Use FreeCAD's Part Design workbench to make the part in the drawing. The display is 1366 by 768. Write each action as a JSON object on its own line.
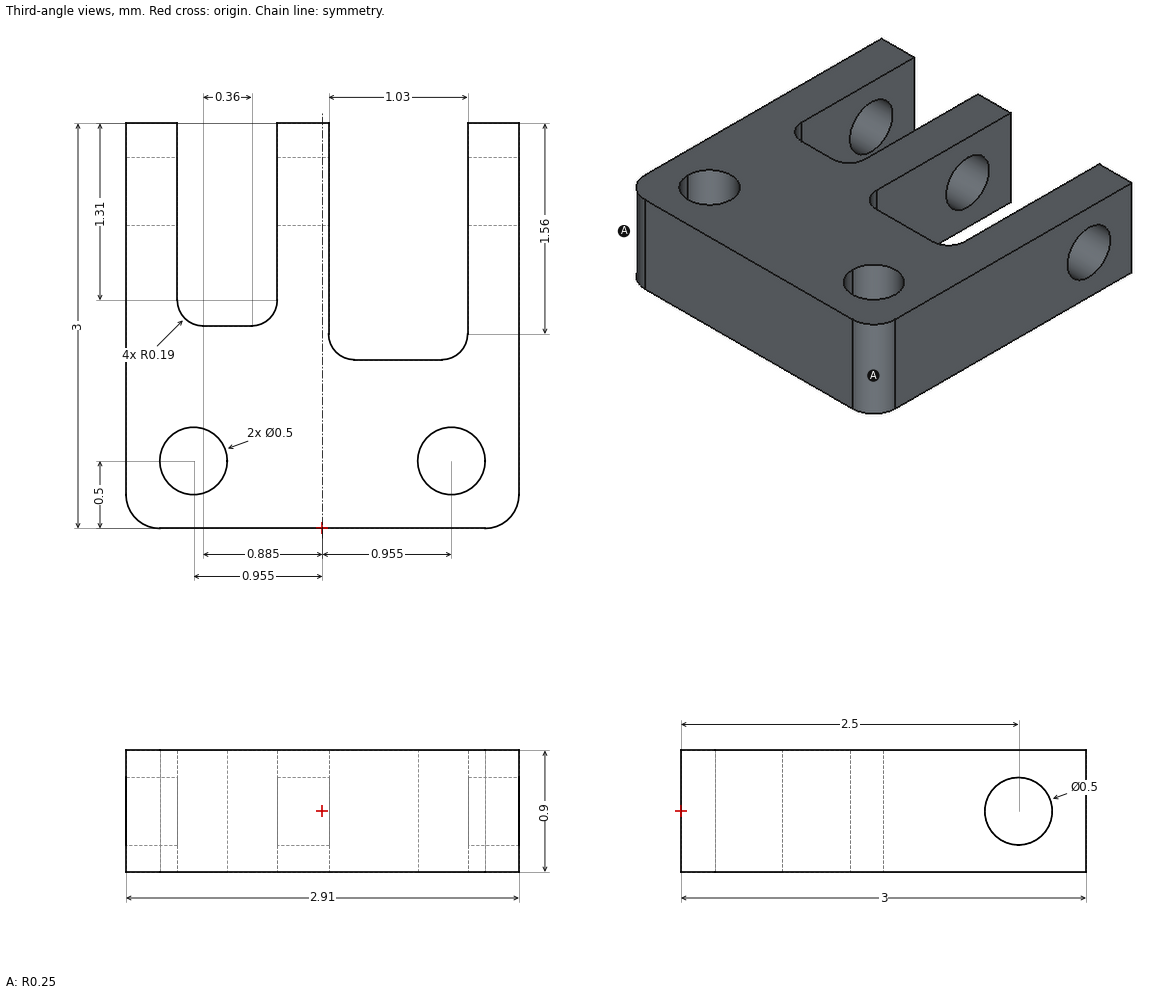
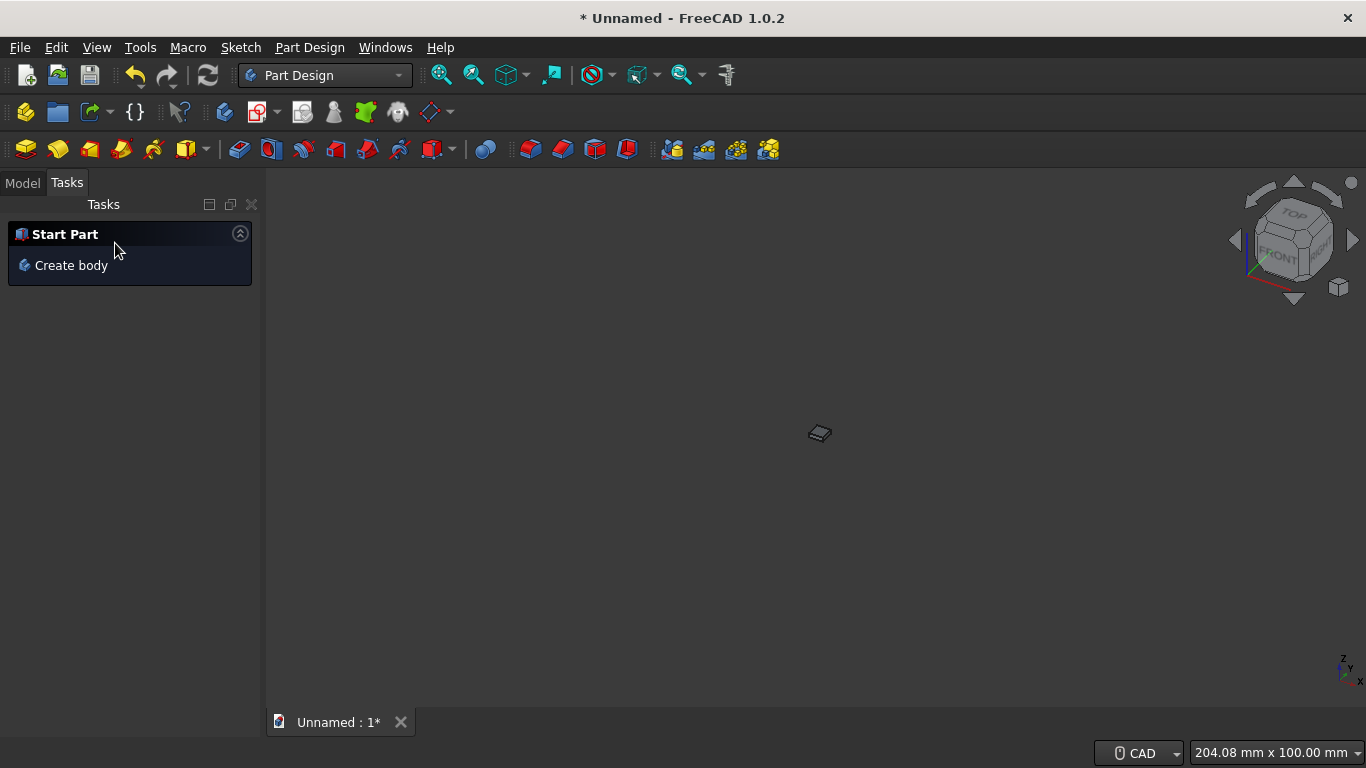
{"action": "key", "text": "v f"}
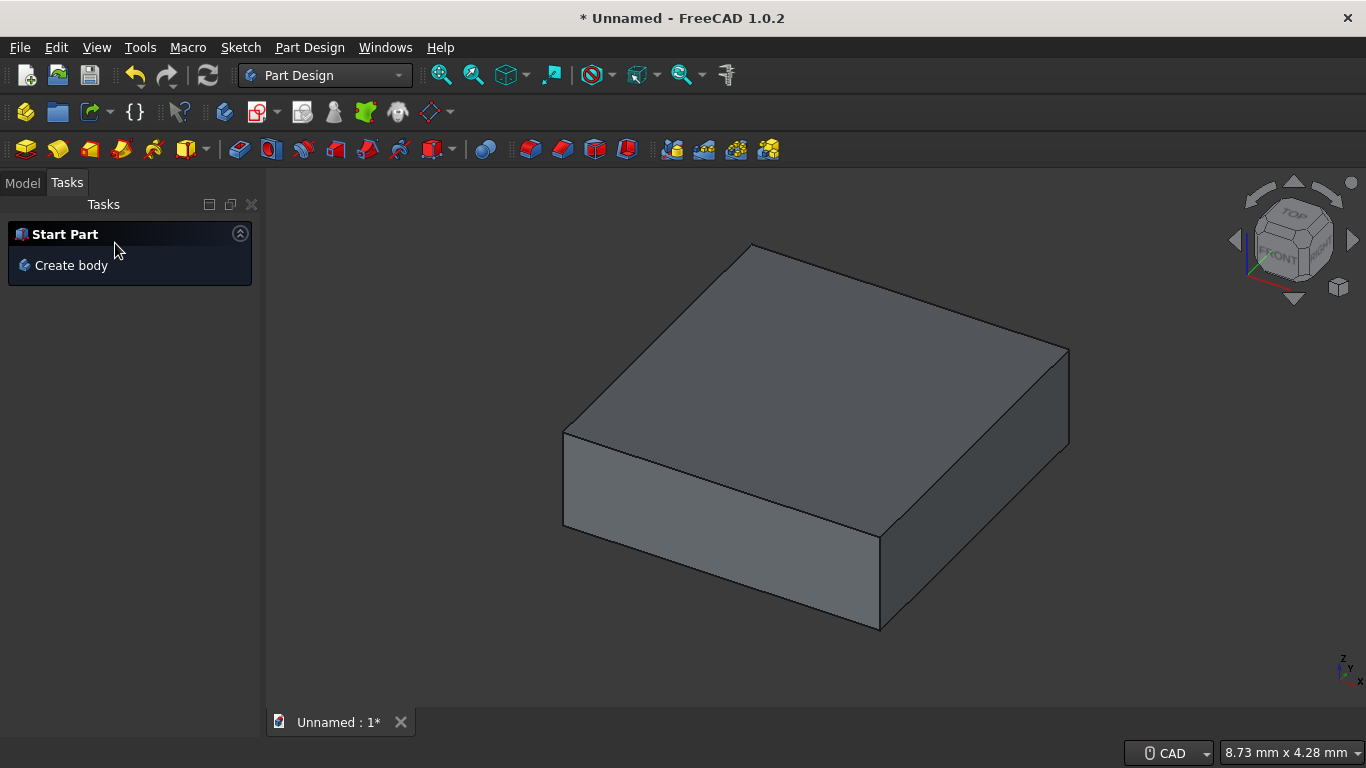
{"action": "left_click", "coordinate": [880, 583]}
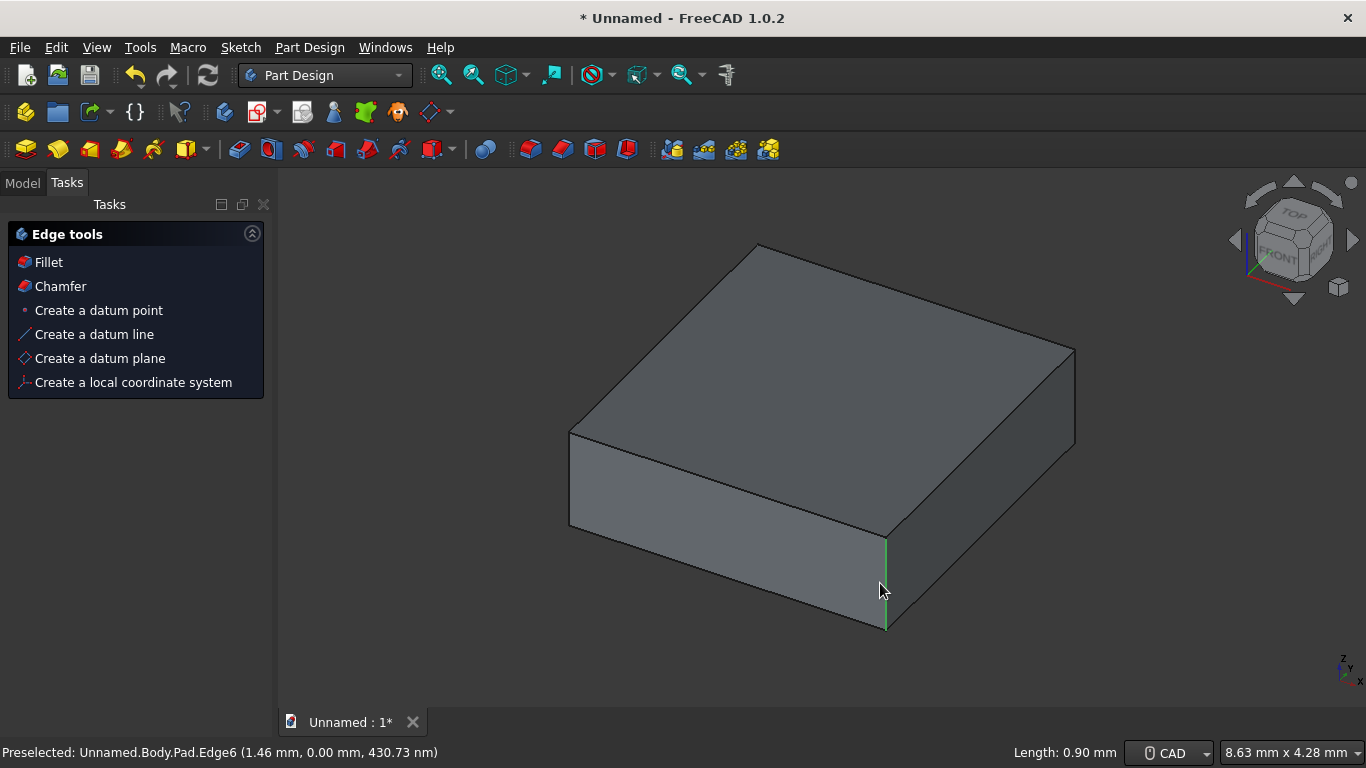
{"action": "key", "text": "0"}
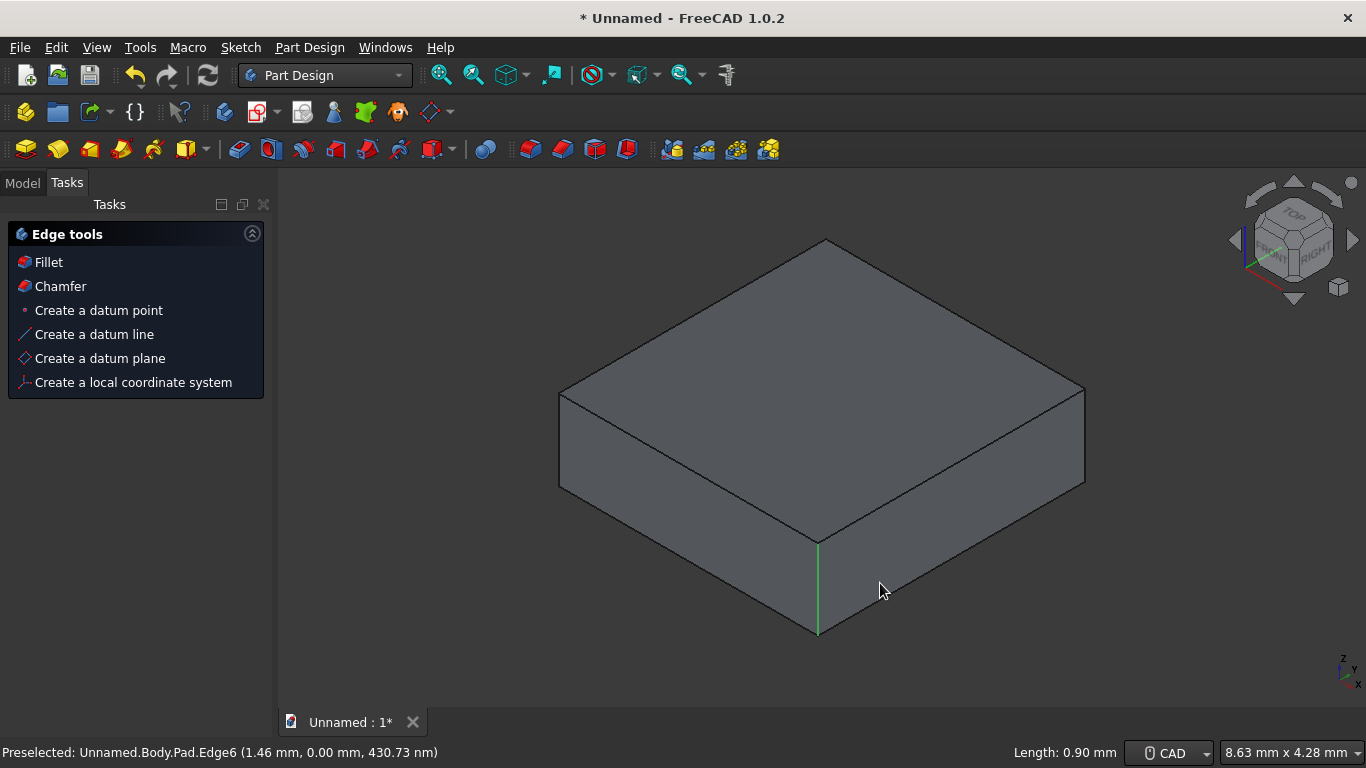
{"action": "key", "text": "2"}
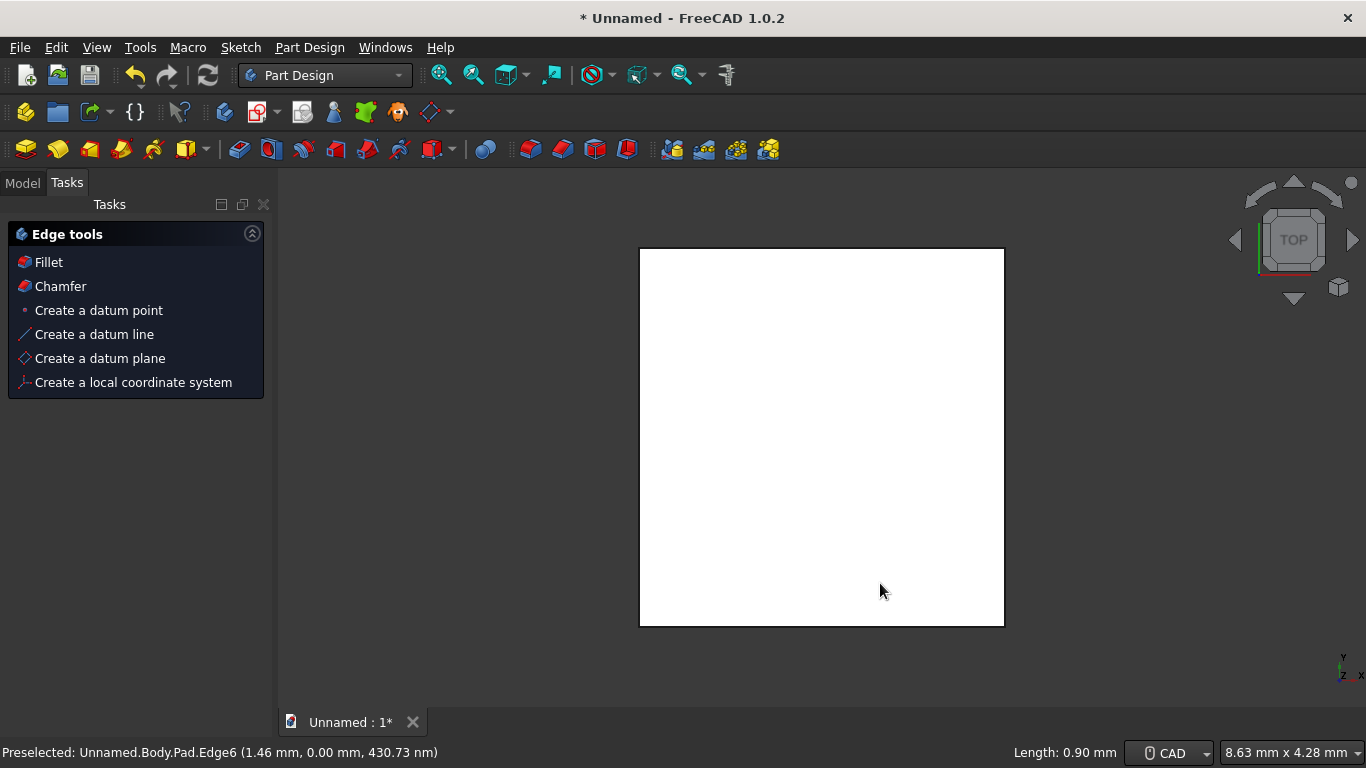
{"action": "key", "text": "1"}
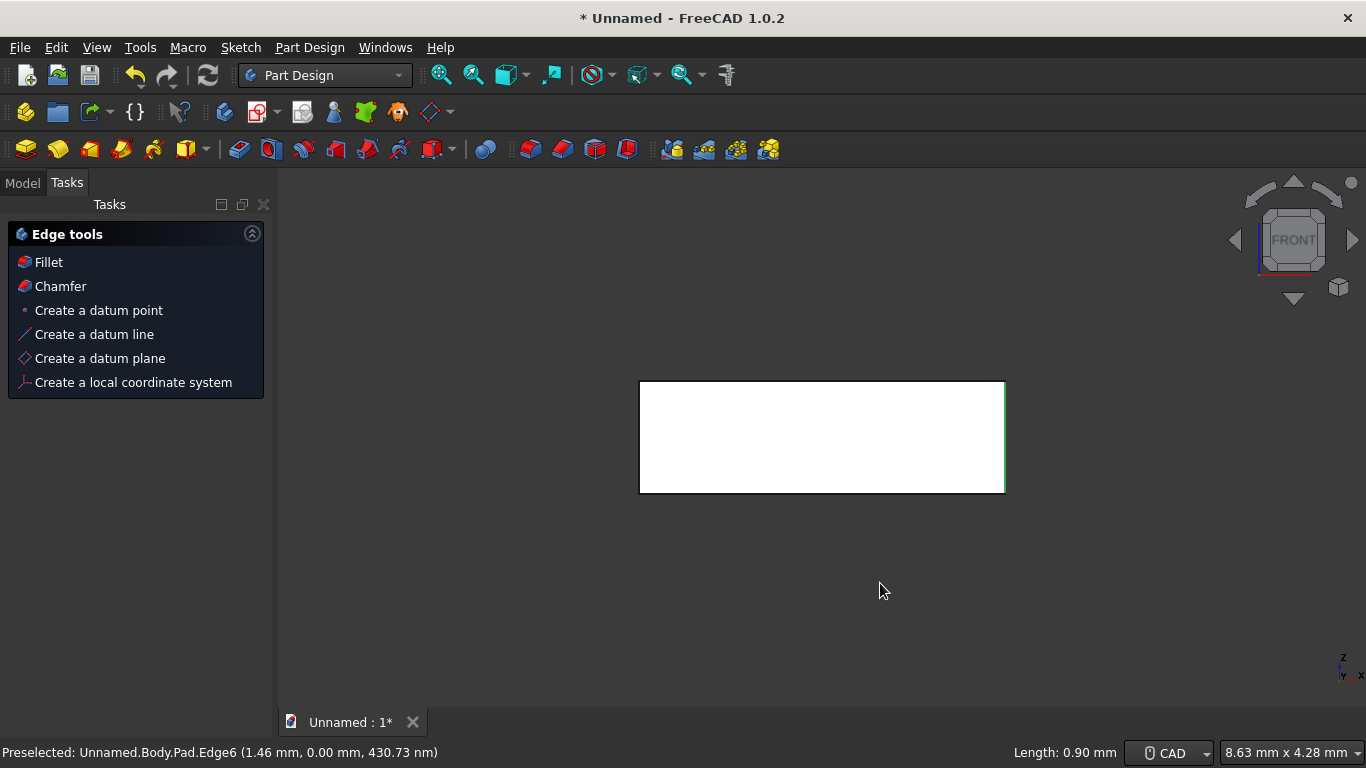
{"action": "key", "text": "v f"}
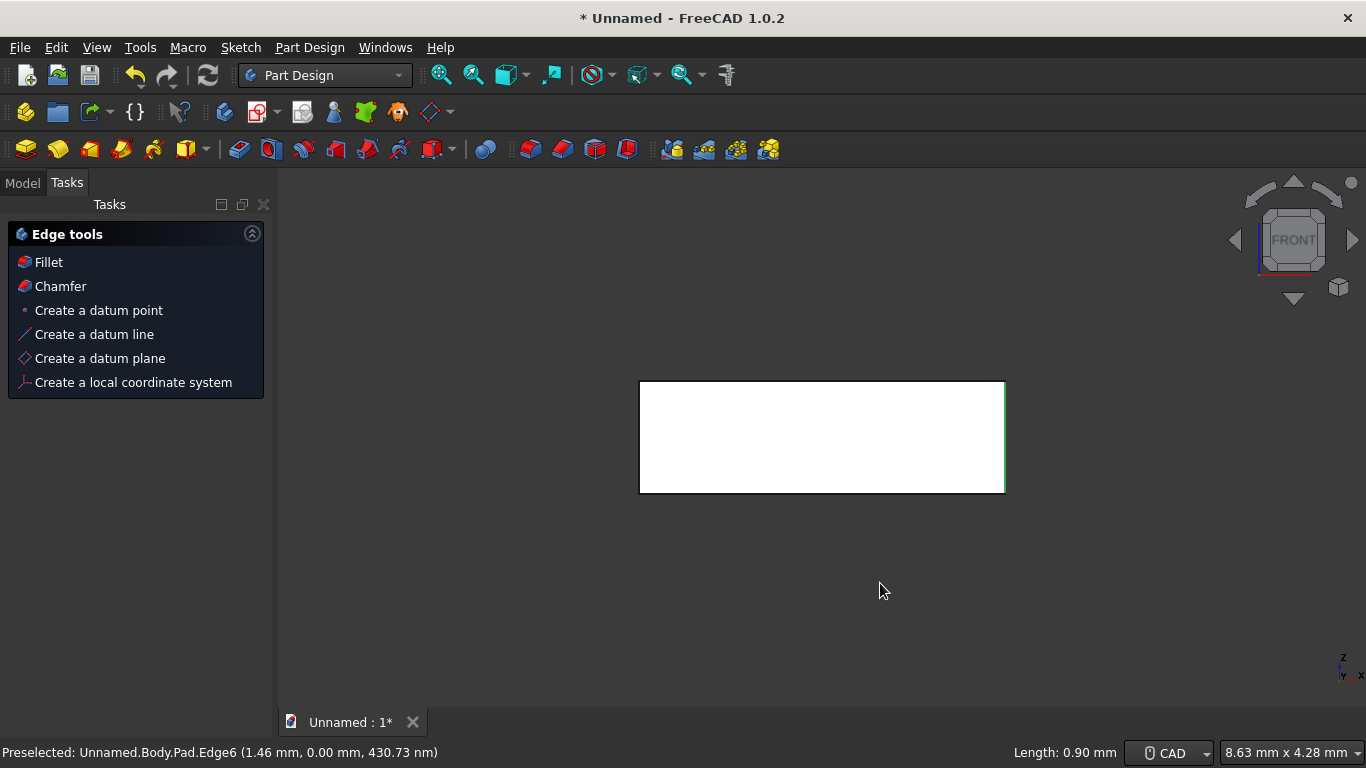
{"action": "left_click", "coordinate": [639, 437], "text": "ctrl"}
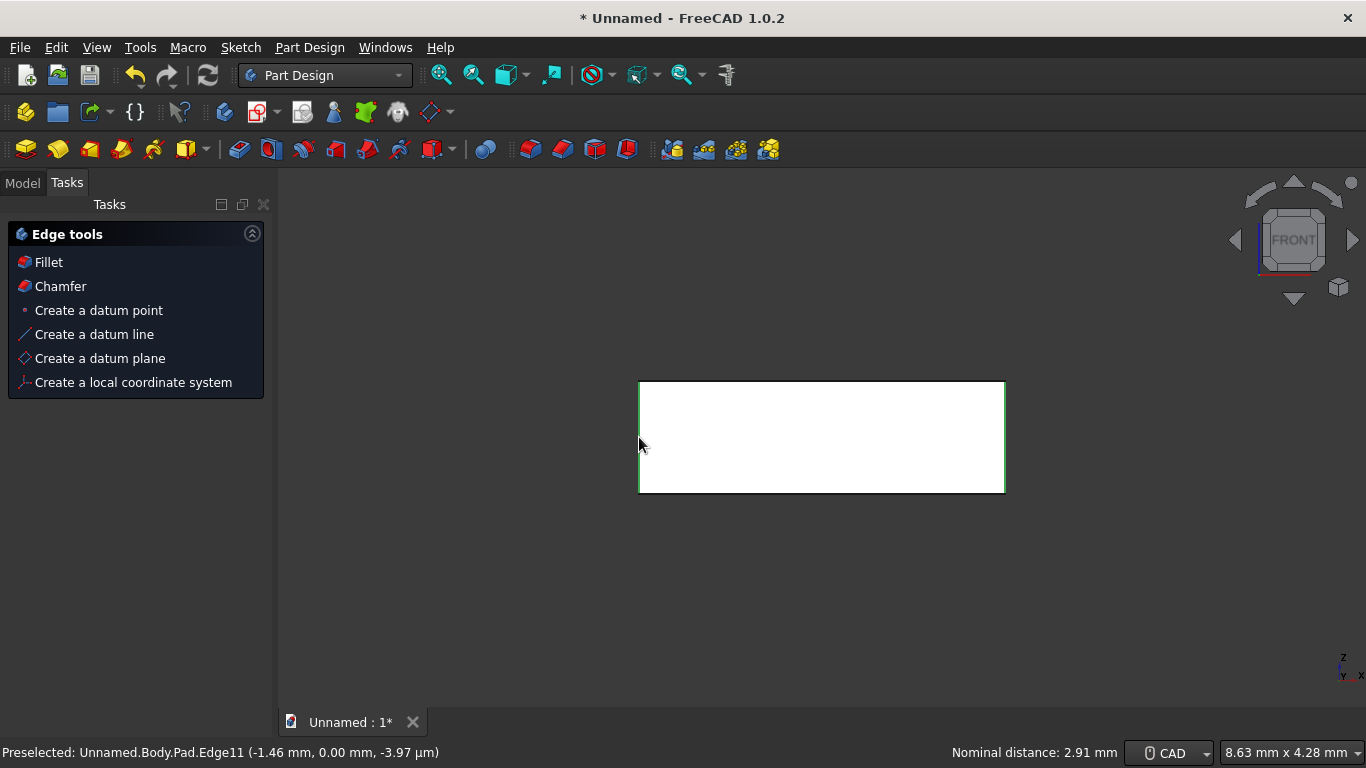
{"action": "left_click", "coordinate": [532, 150]}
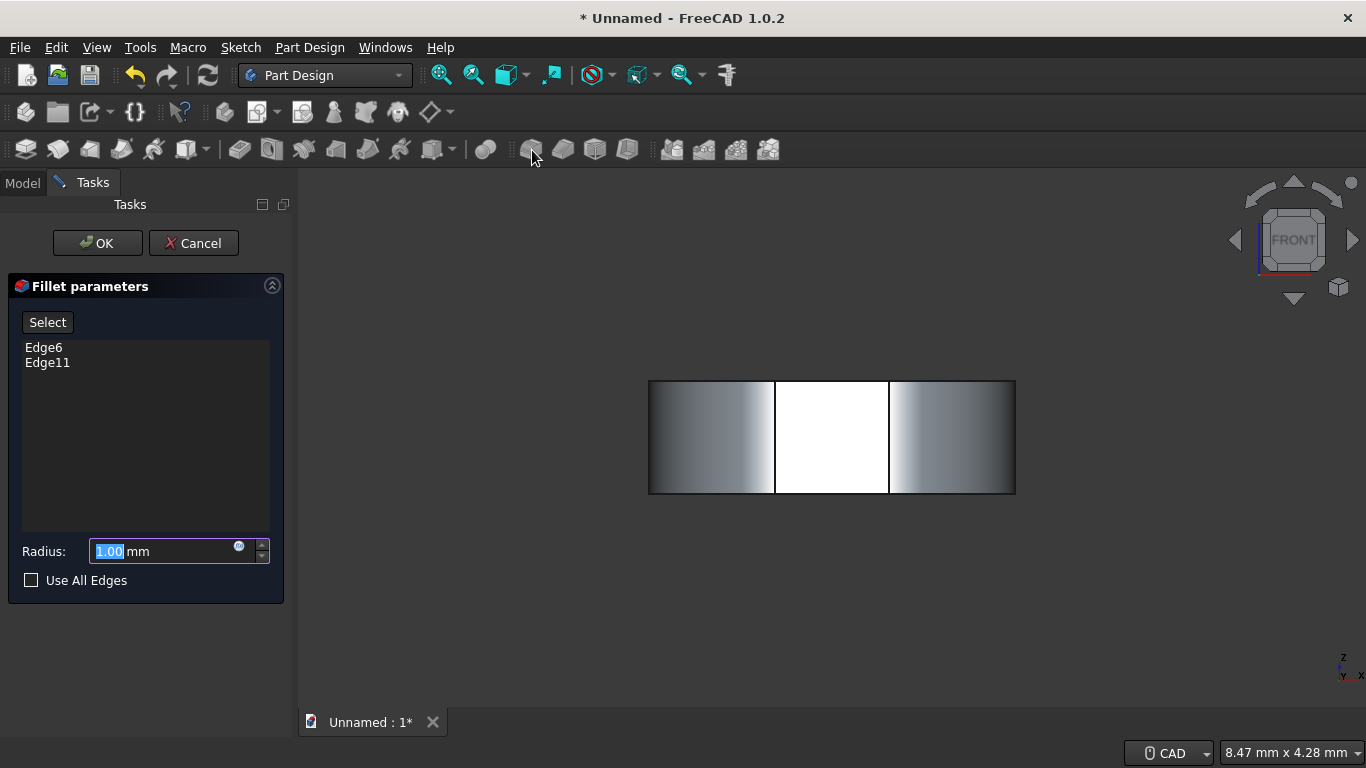
{"action": "type", "text": "0.25"}
{"action": "key", "text": "Tab"}